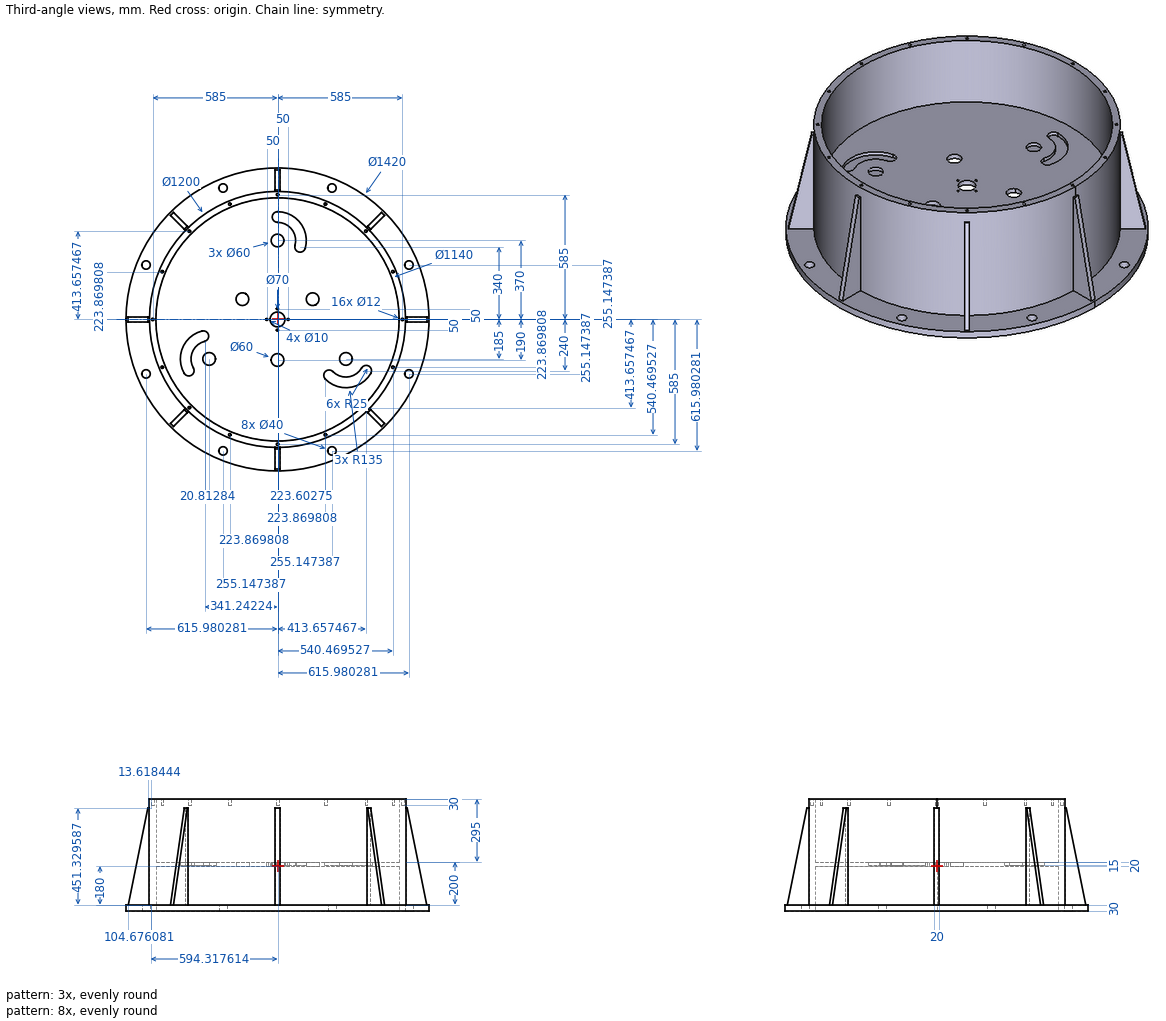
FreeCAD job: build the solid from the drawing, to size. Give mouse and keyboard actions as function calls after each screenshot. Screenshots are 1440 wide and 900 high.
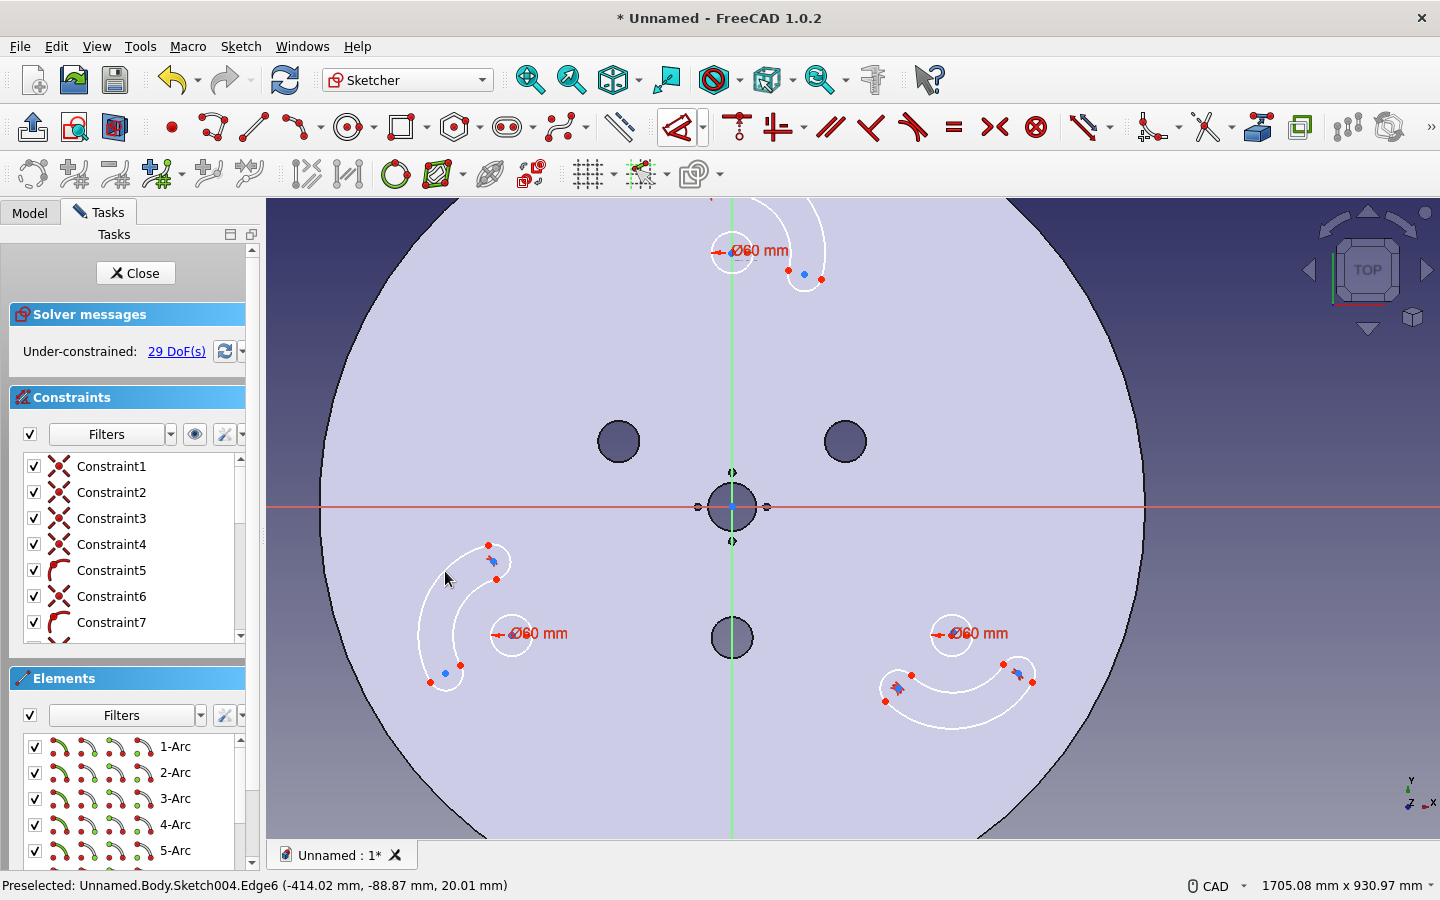
click(509, 569)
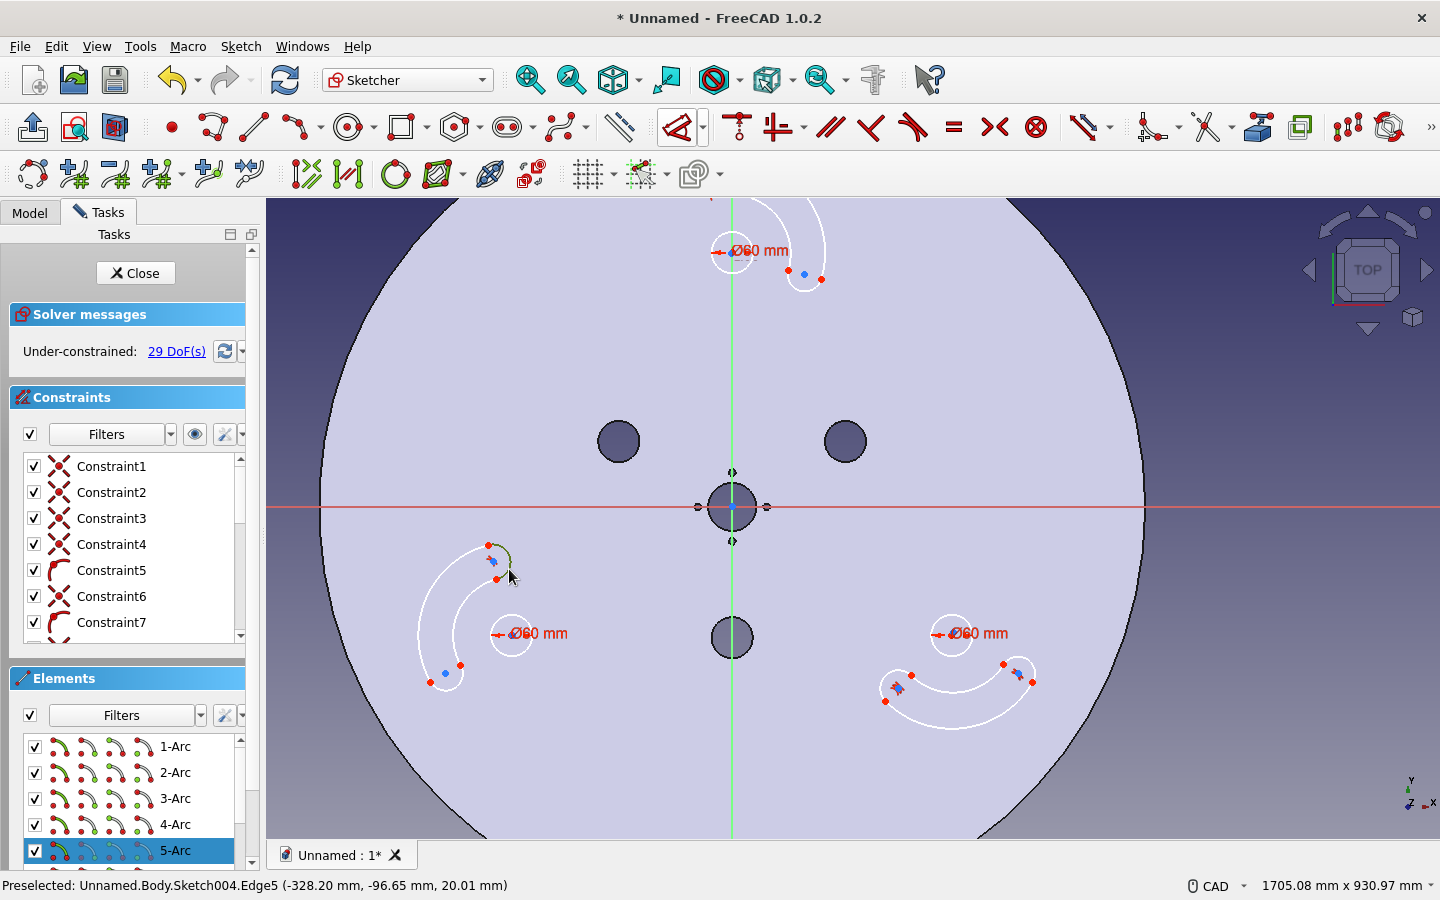
click(469, 595)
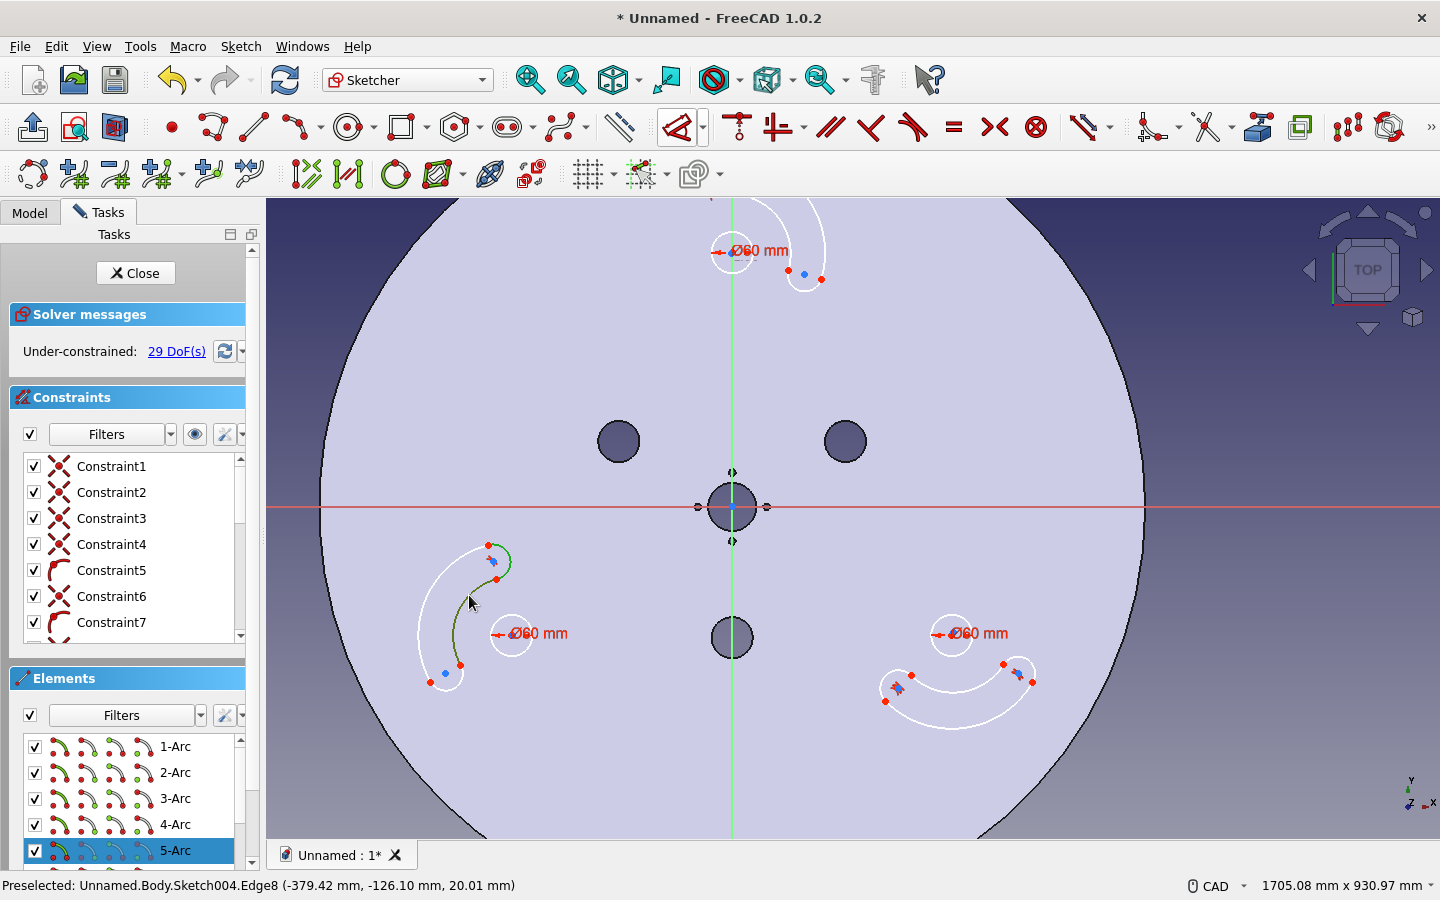
key(t)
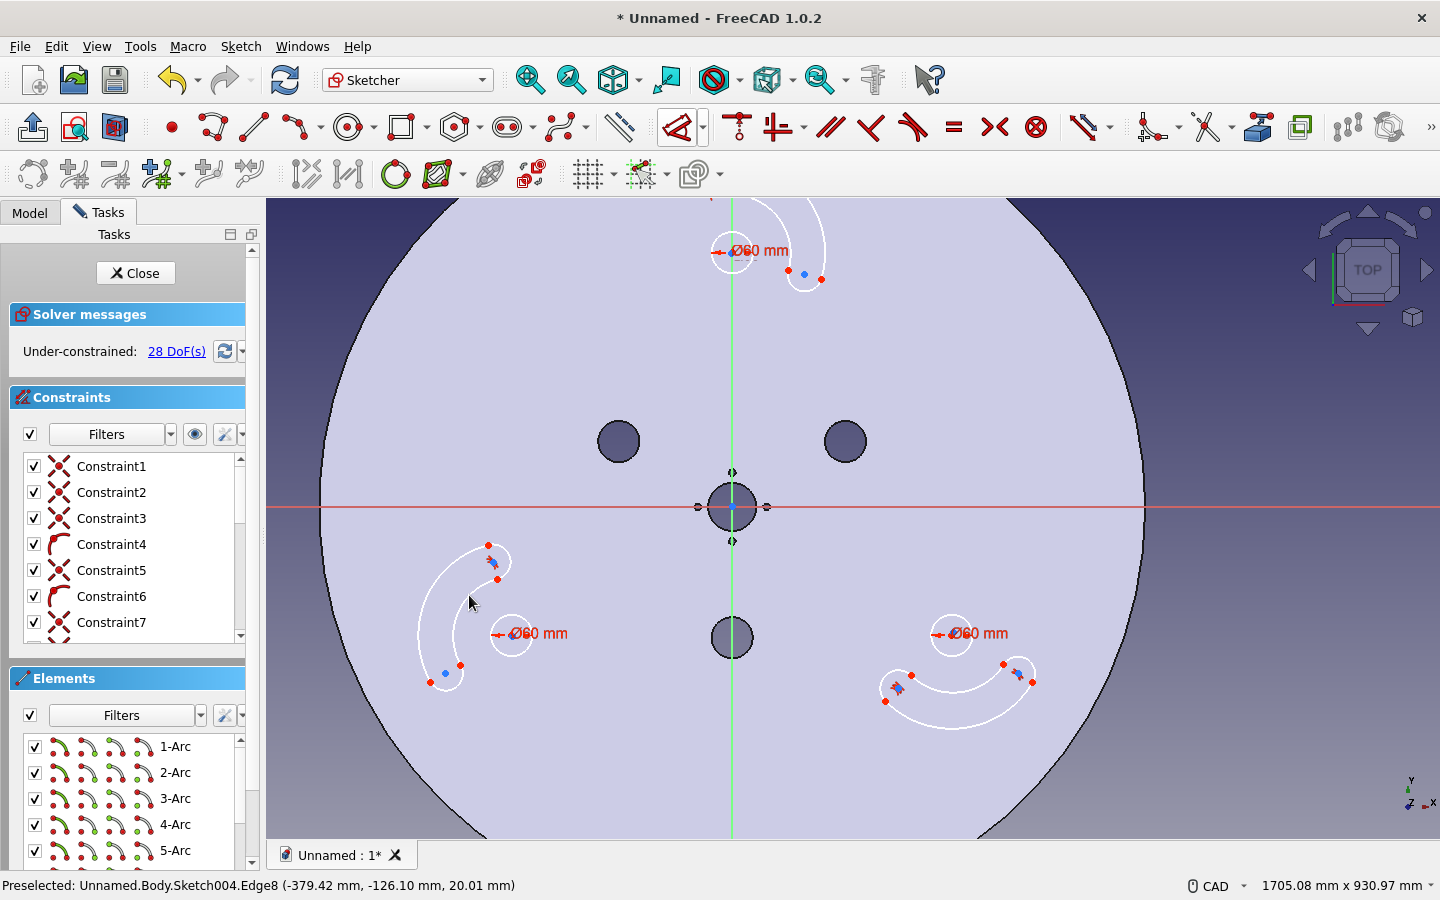
click(445, 571)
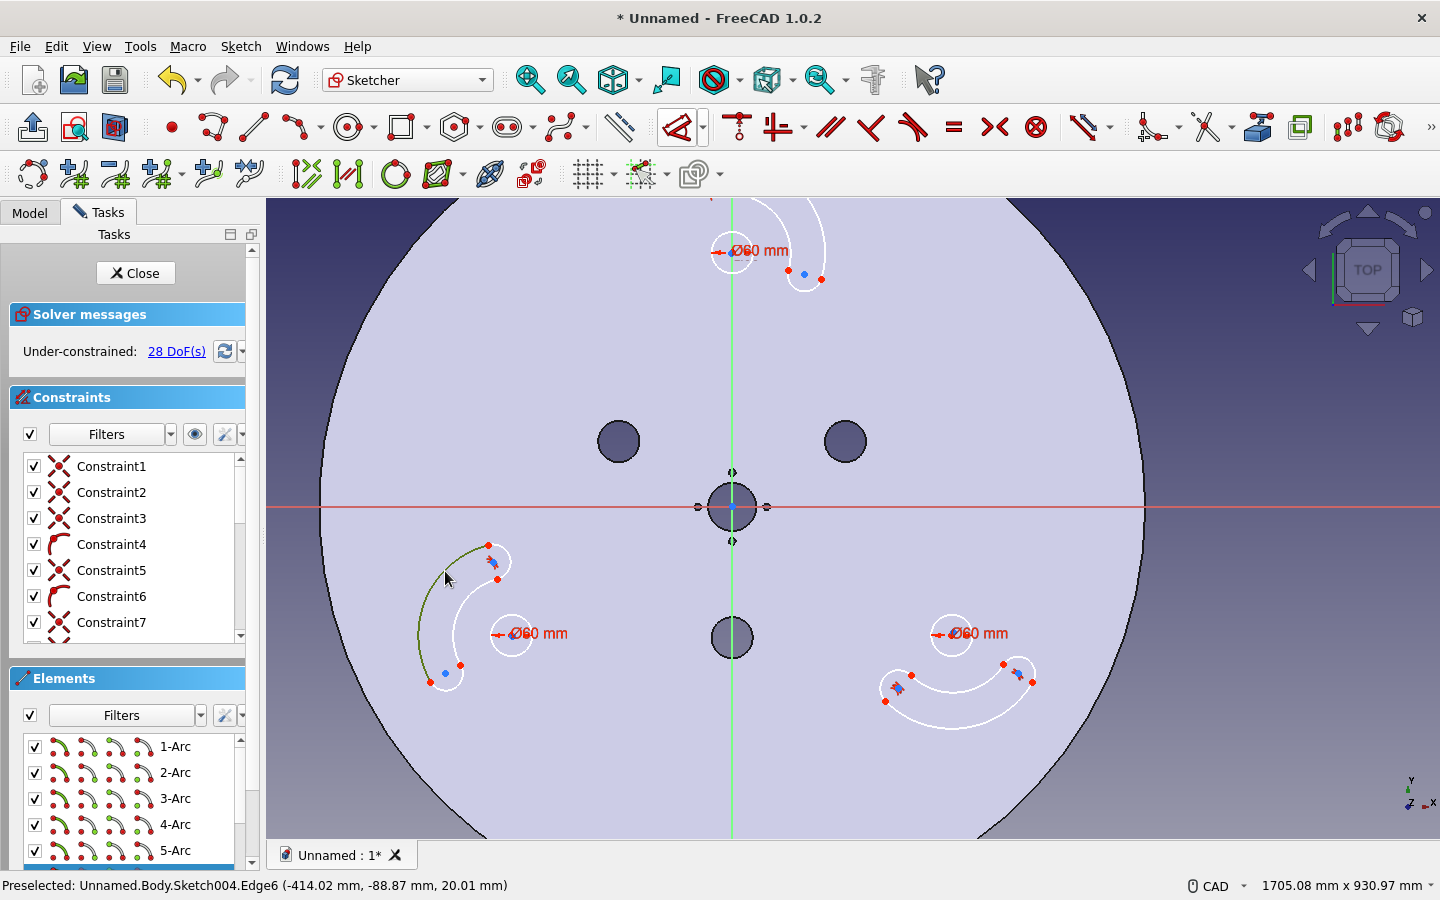
click(444, 691)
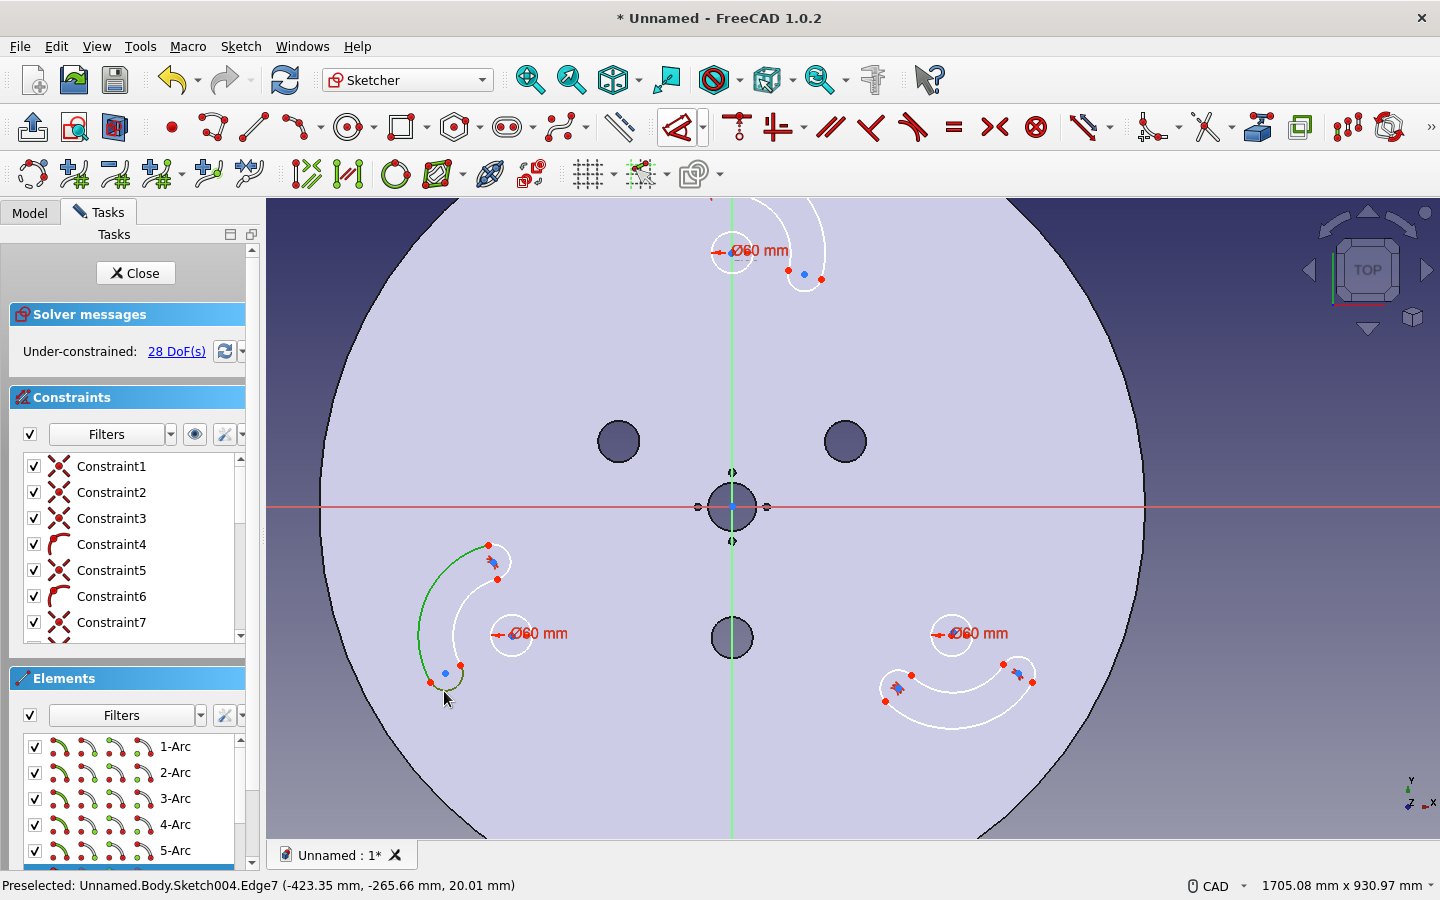
key(t)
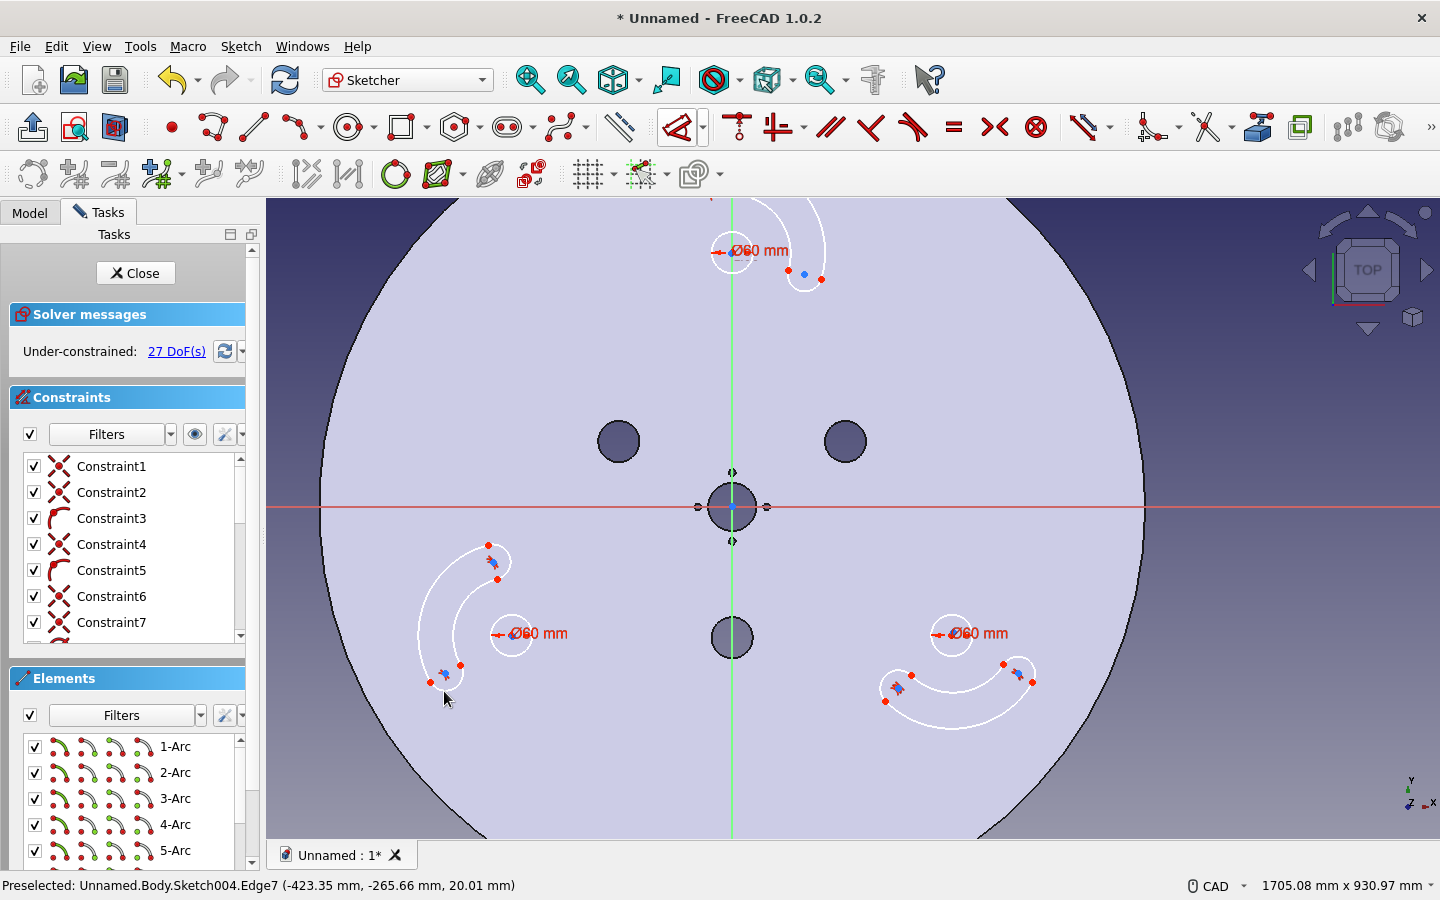
click(444, 691)